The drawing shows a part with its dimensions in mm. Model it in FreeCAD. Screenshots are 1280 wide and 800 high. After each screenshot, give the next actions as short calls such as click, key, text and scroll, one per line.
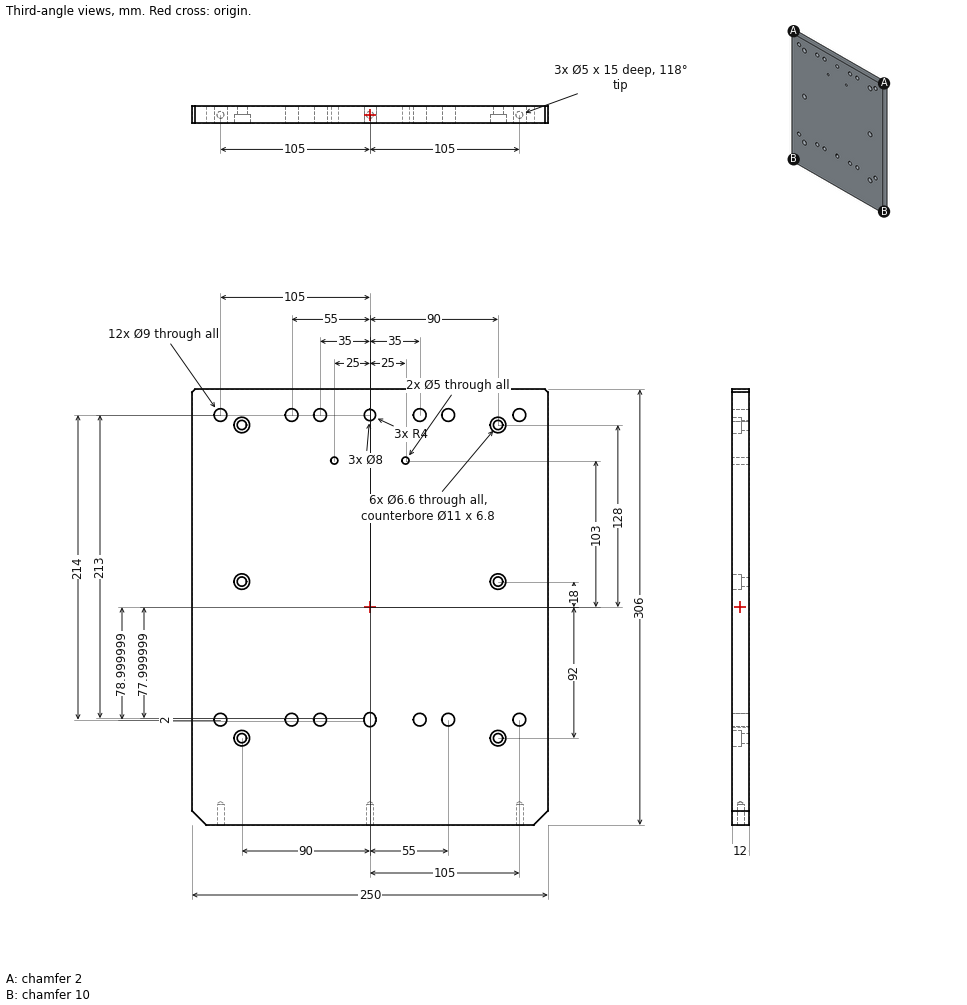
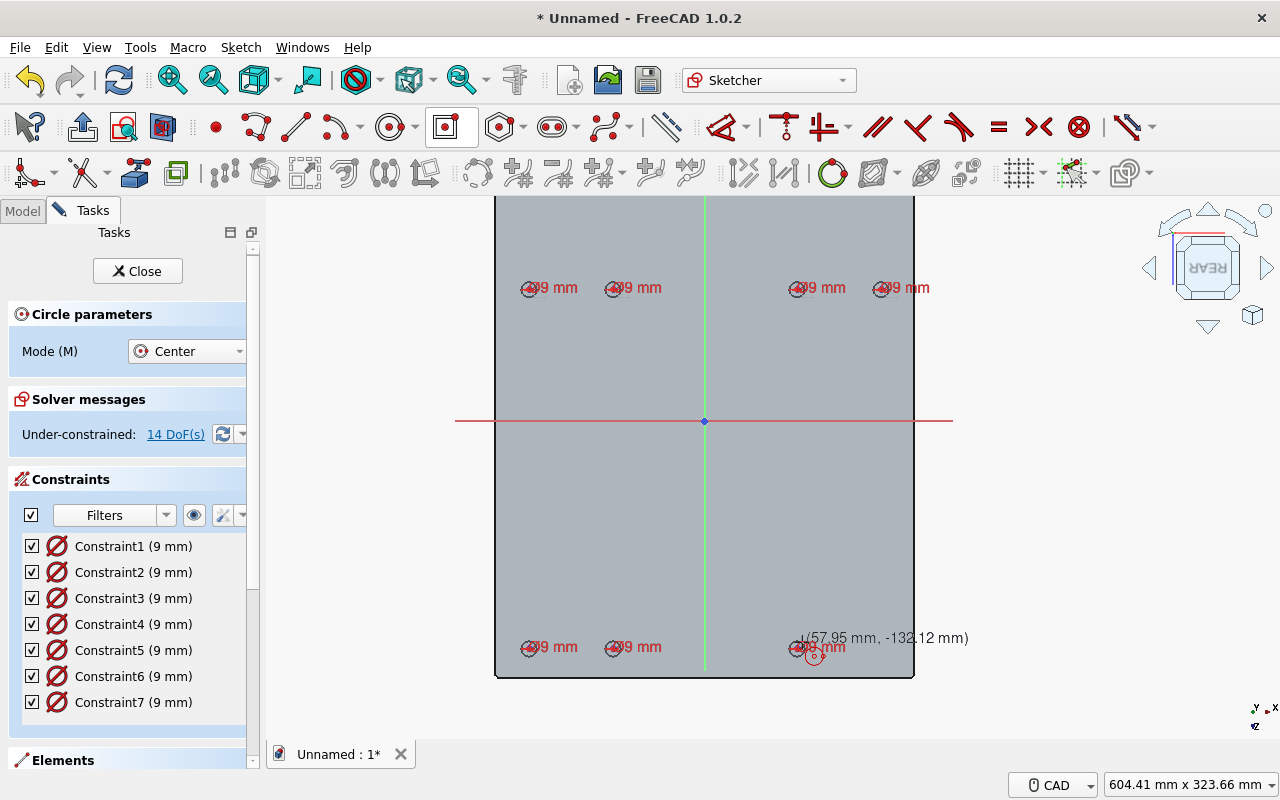
scroll(881, 648, up, 6)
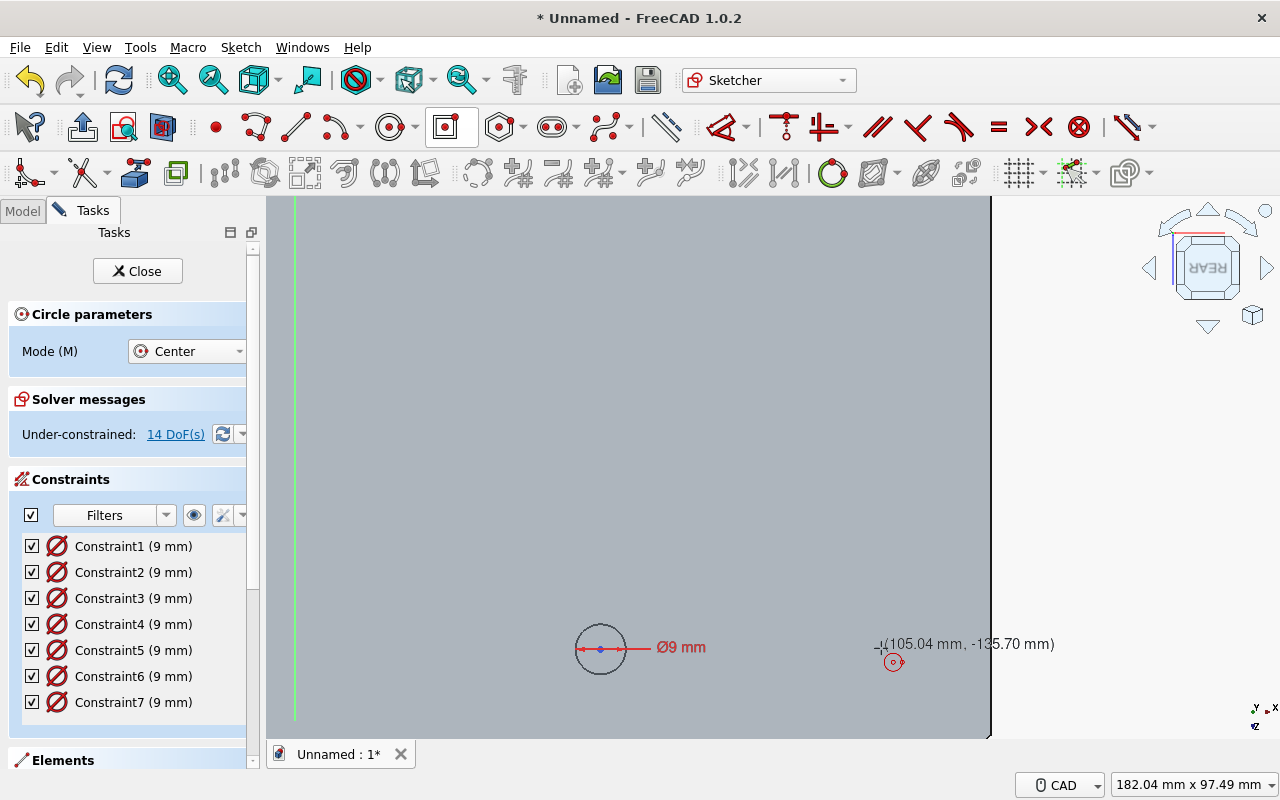
scroll(881, 648, down, 6)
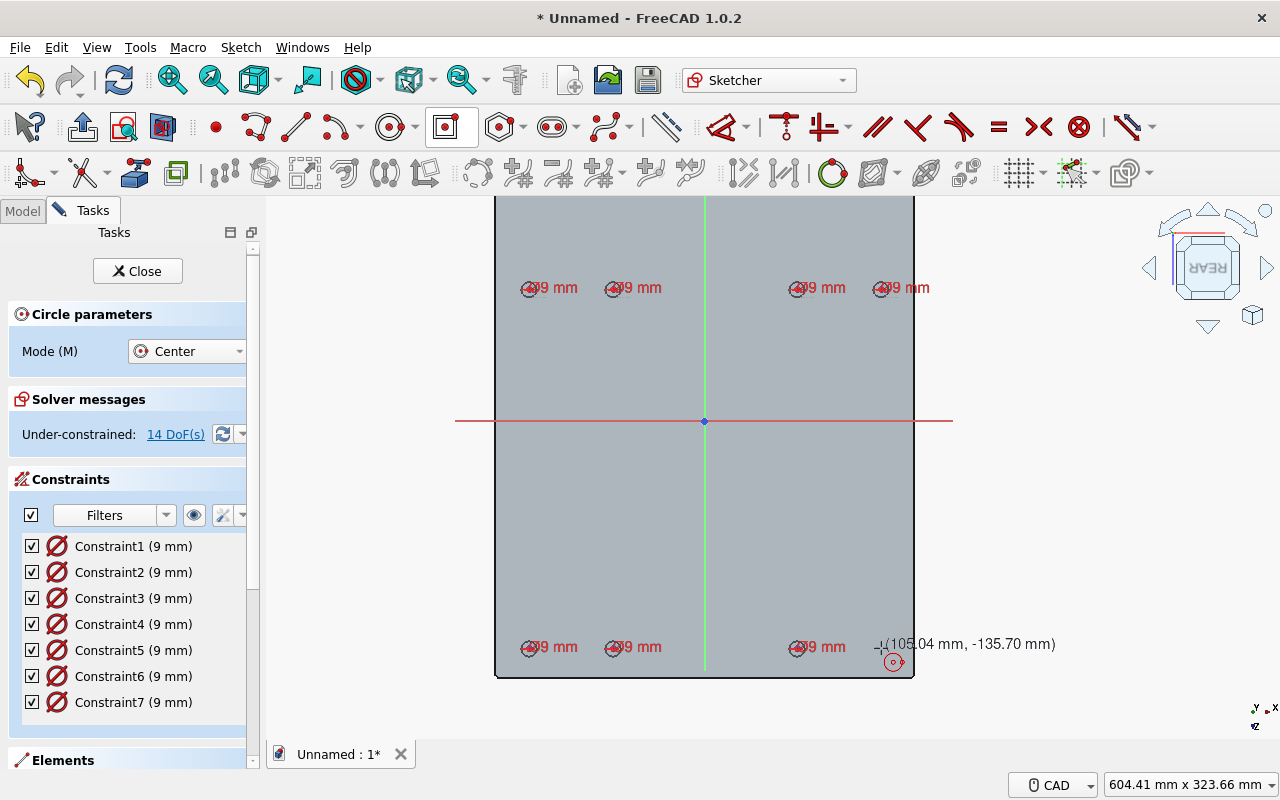
click(881, 648)
move(886, 642)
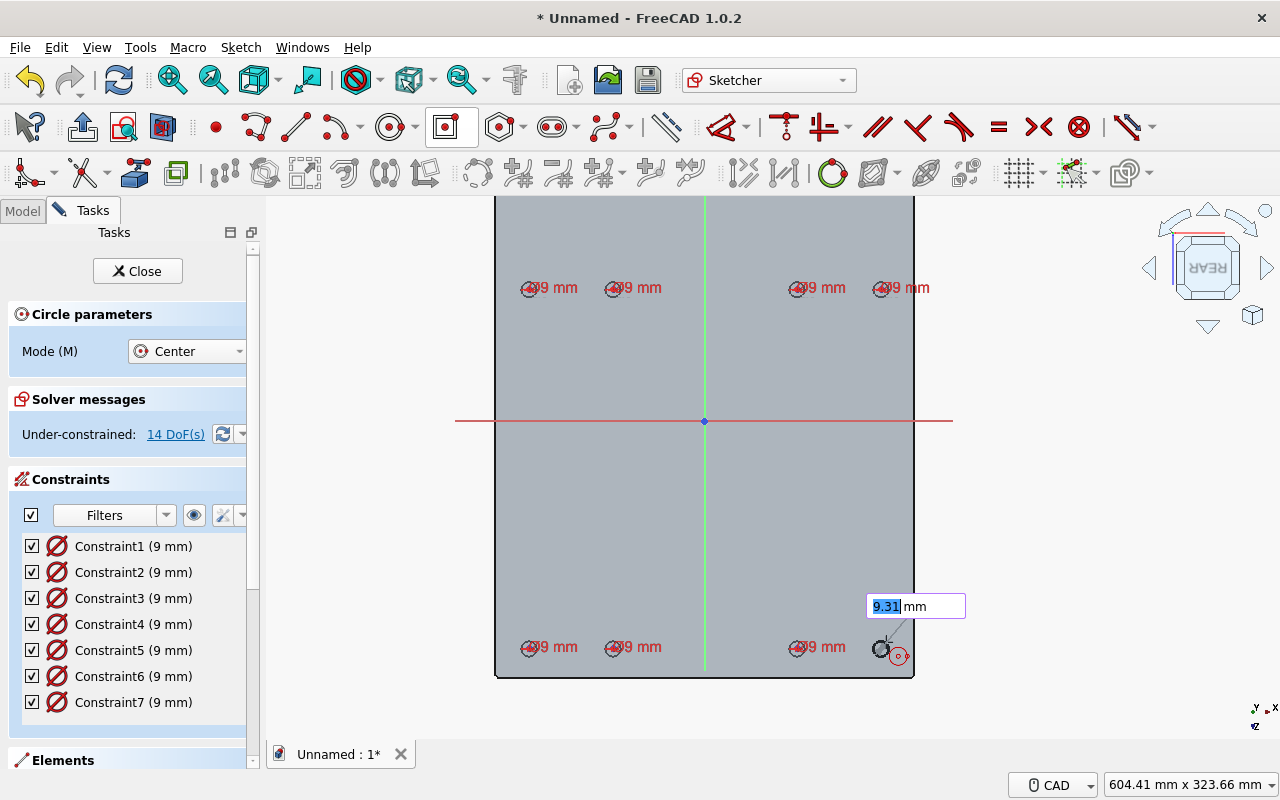
text(9)
key(Return)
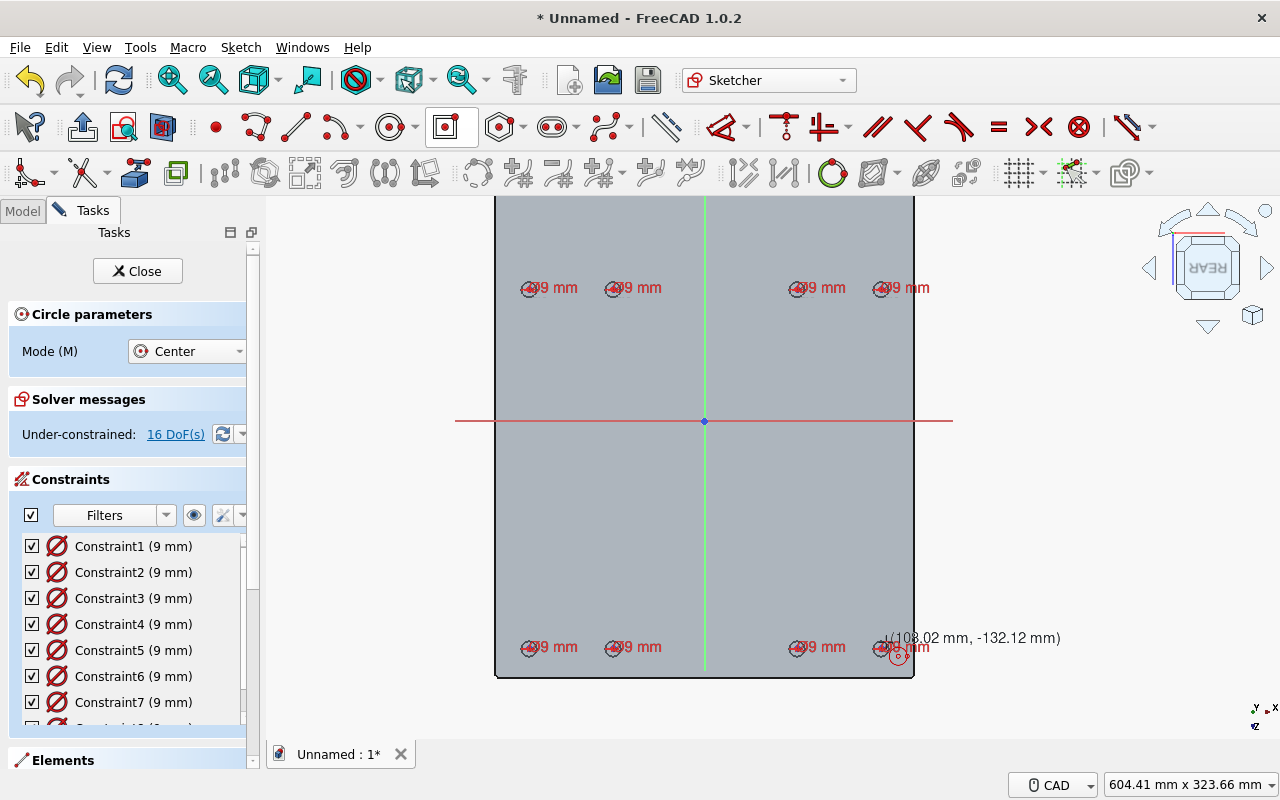
scroll(646, 648, up, 6)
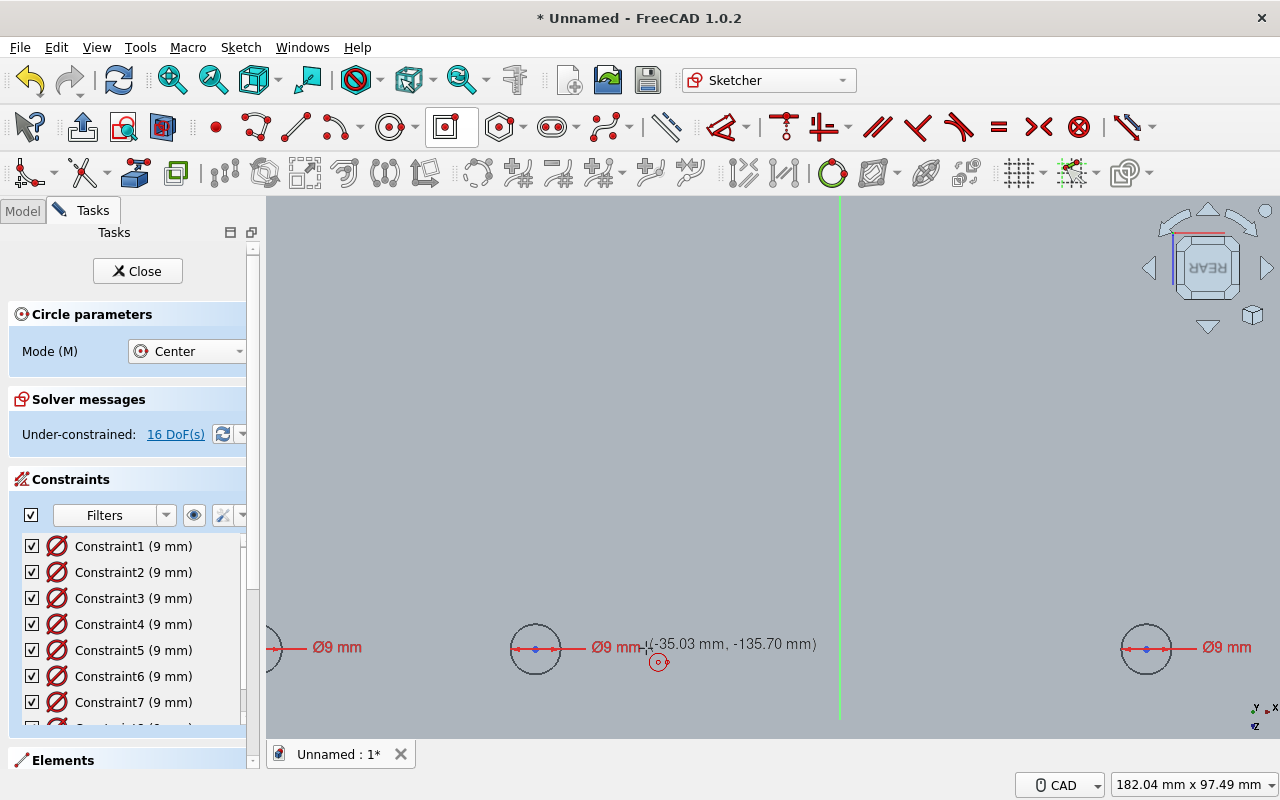
scroll(646, 648, down, 6)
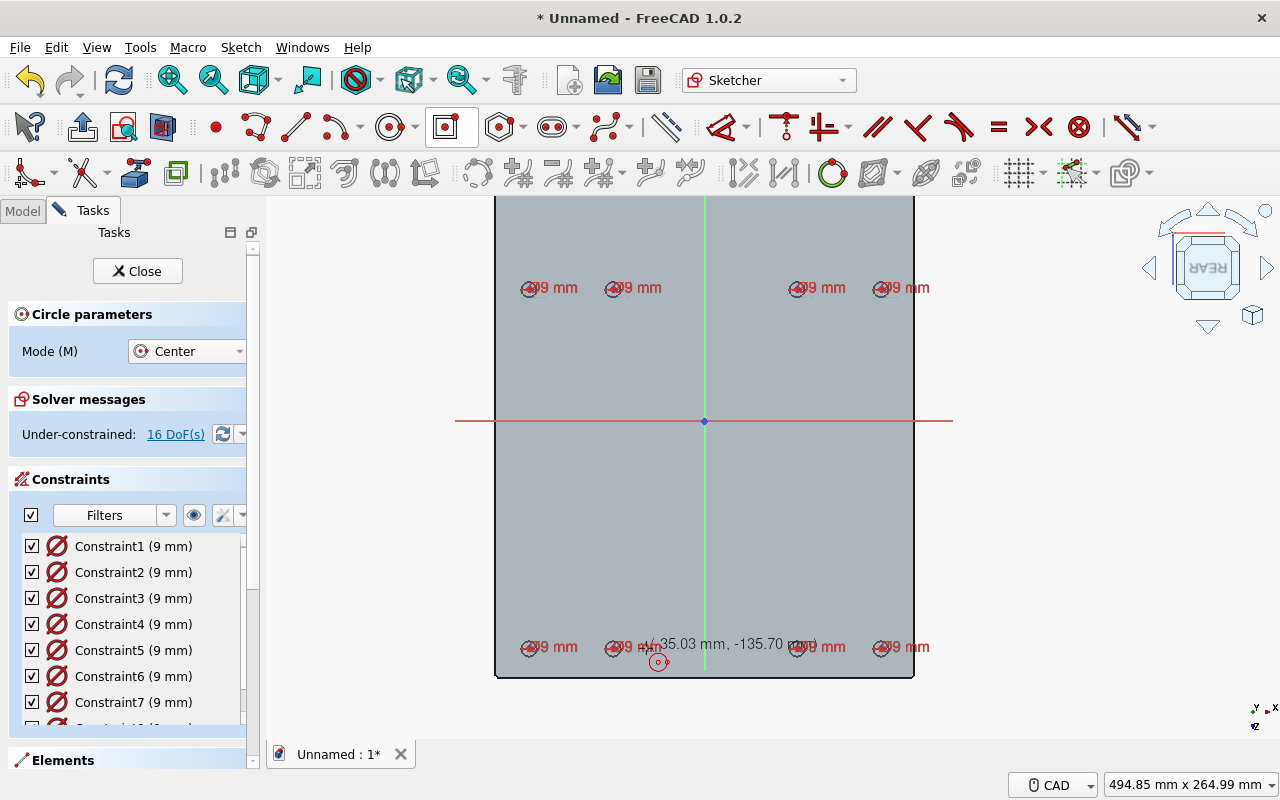
click(646, 648)
move(651, 642)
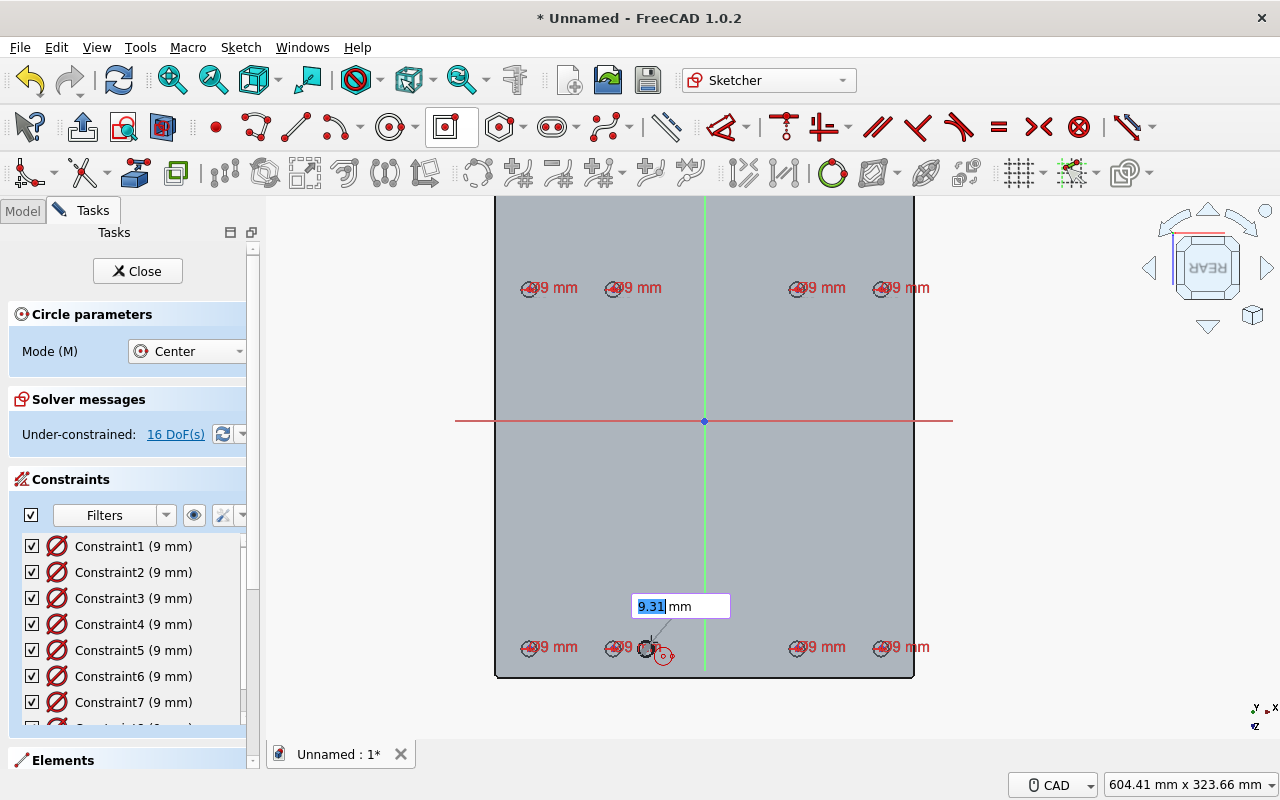
text(9)
key(Return)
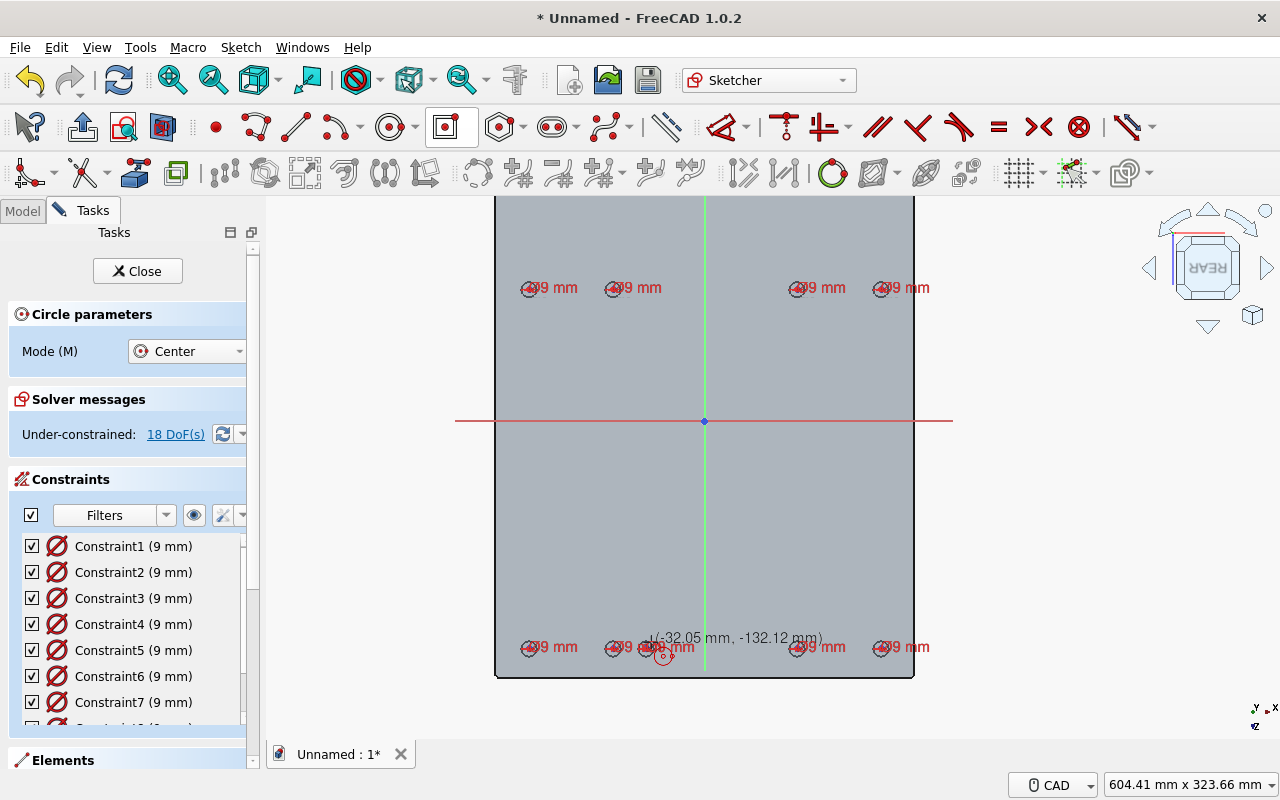
scroll(763, 648, up, 6)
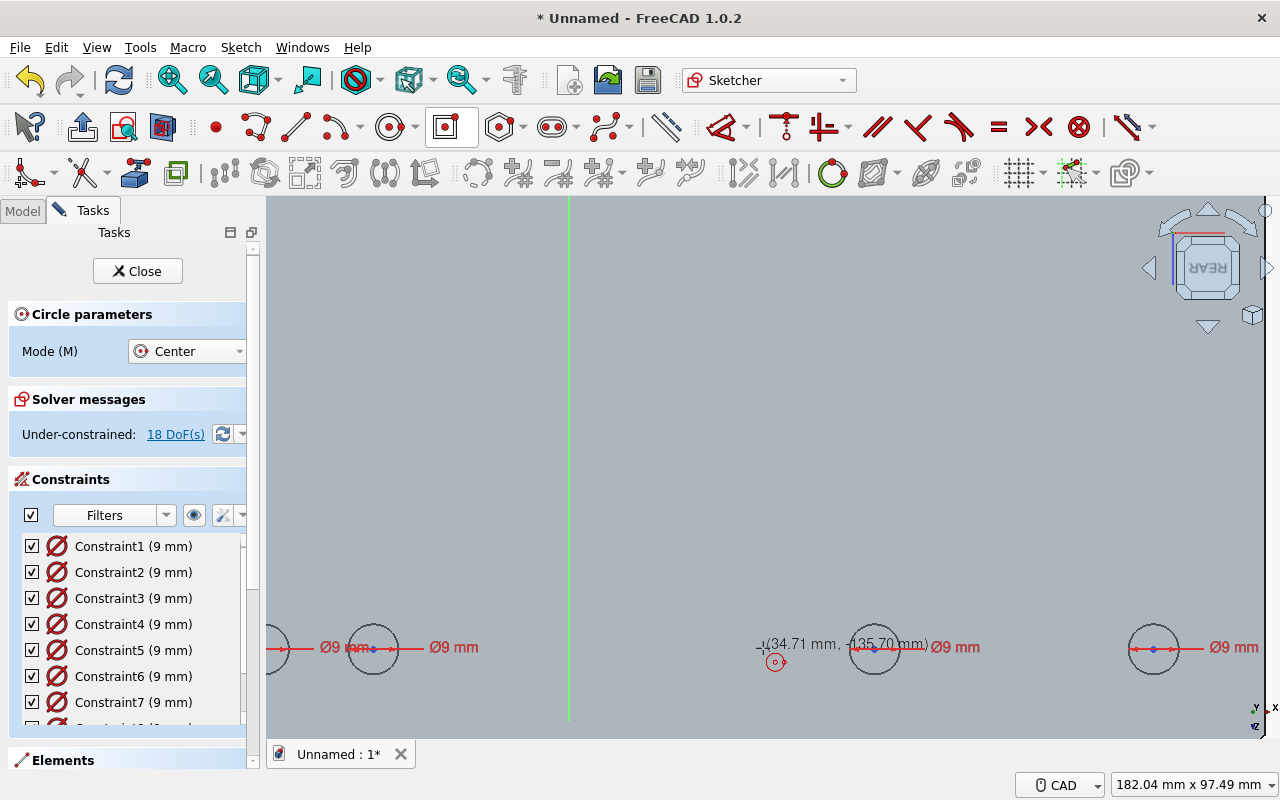
scroll(763, 648, down, 6)